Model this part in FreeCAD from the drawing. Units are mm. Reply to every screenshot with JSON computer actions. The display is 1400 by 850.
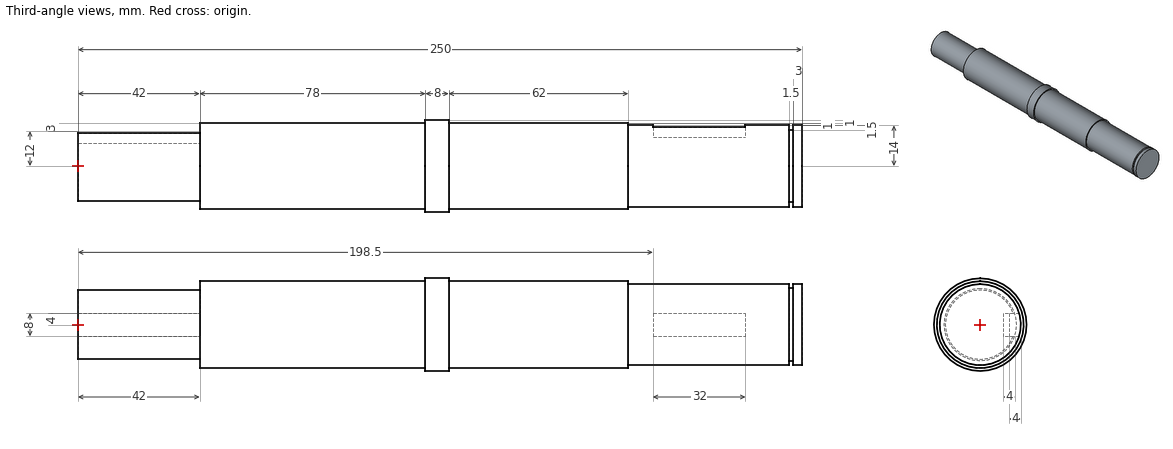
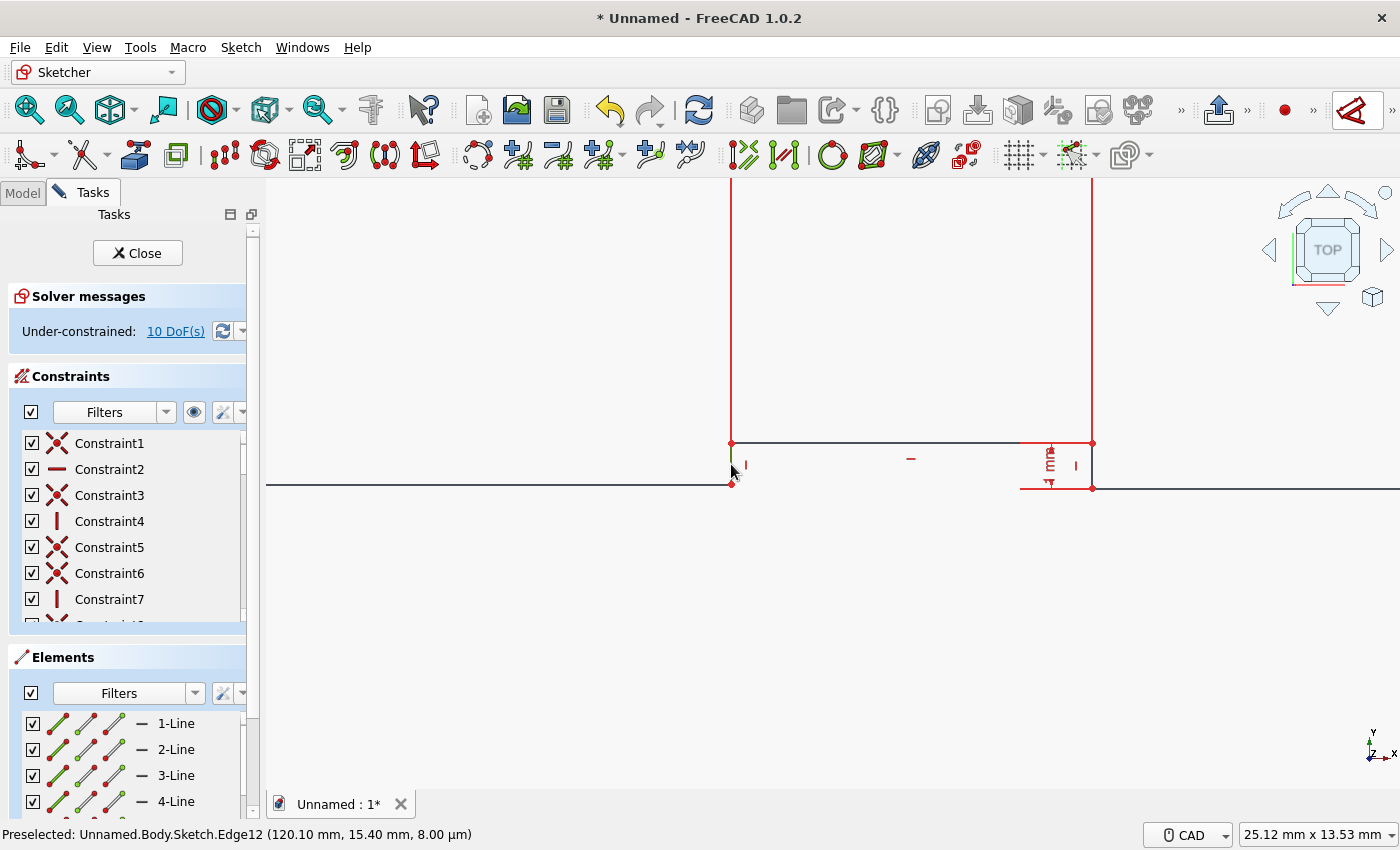
{"action": "left_click", "coordinate": [1378, 110]}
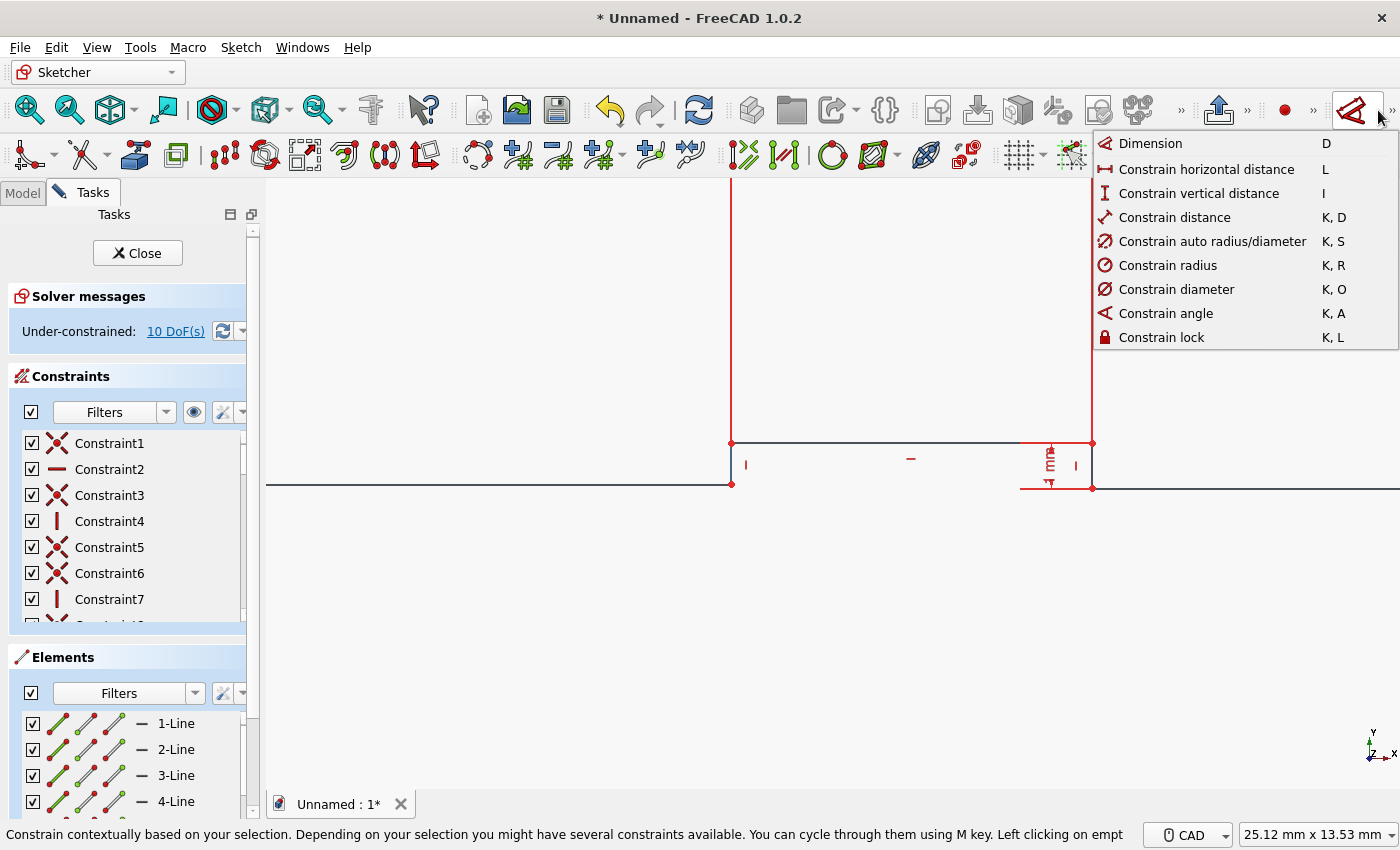
{"action": "left_click", "coordinate": [1246, 193]}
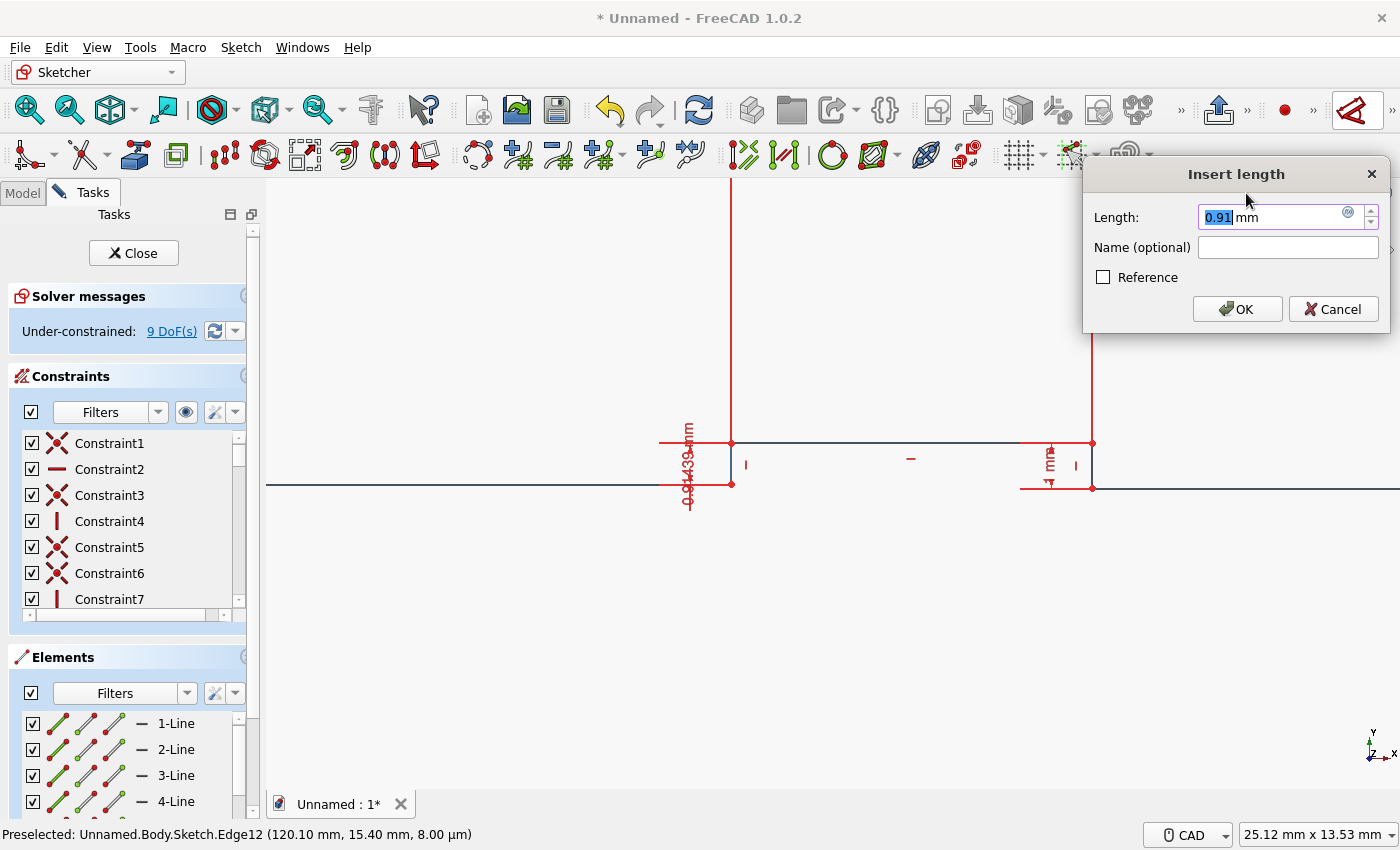
{"action": "type", "text": "1"}
{"action": "key", "text": "Return"}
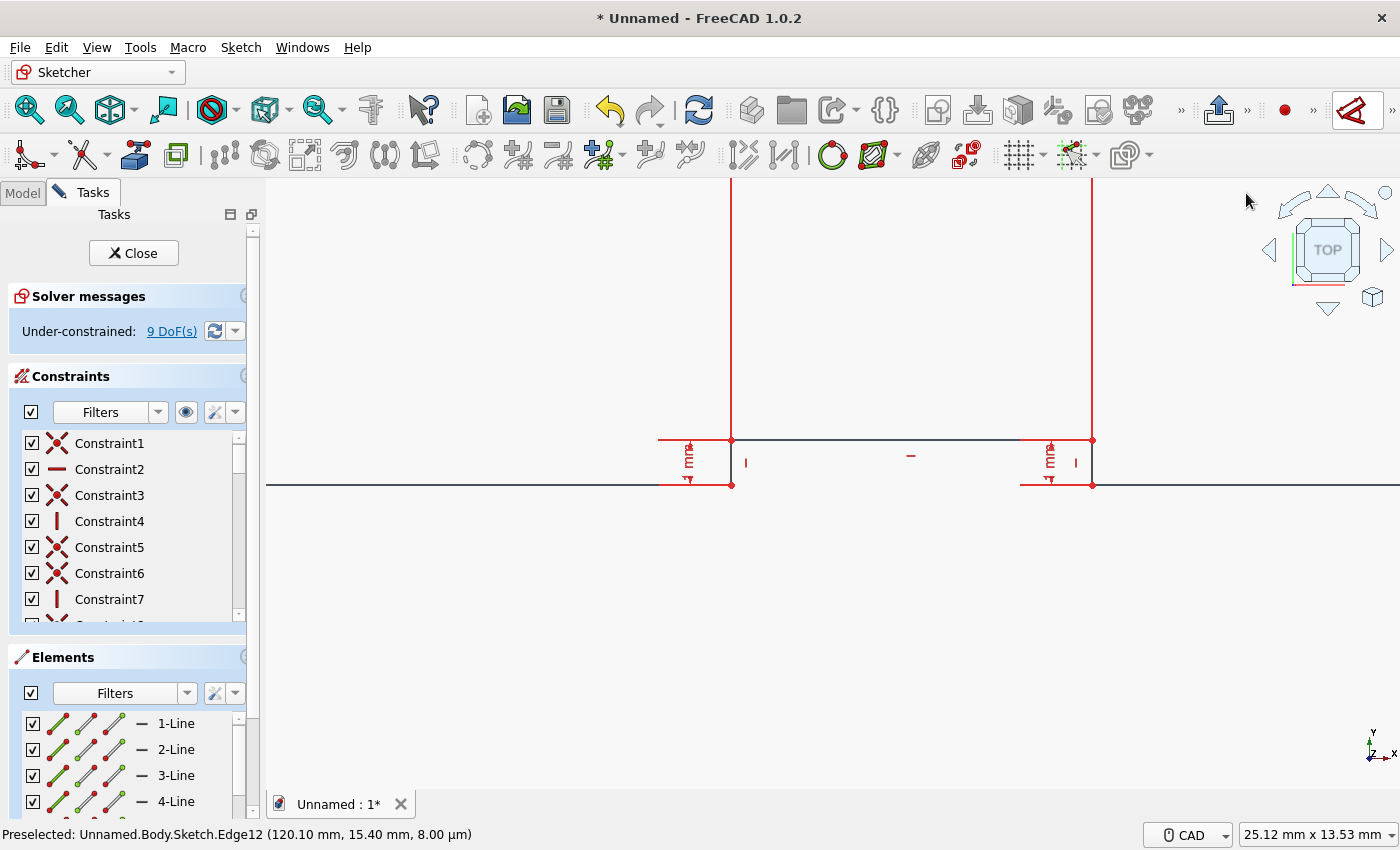
{"action": "scroll", "coordinate": [752, 463], "scroll_direction": "down", "scroll_amount": 14}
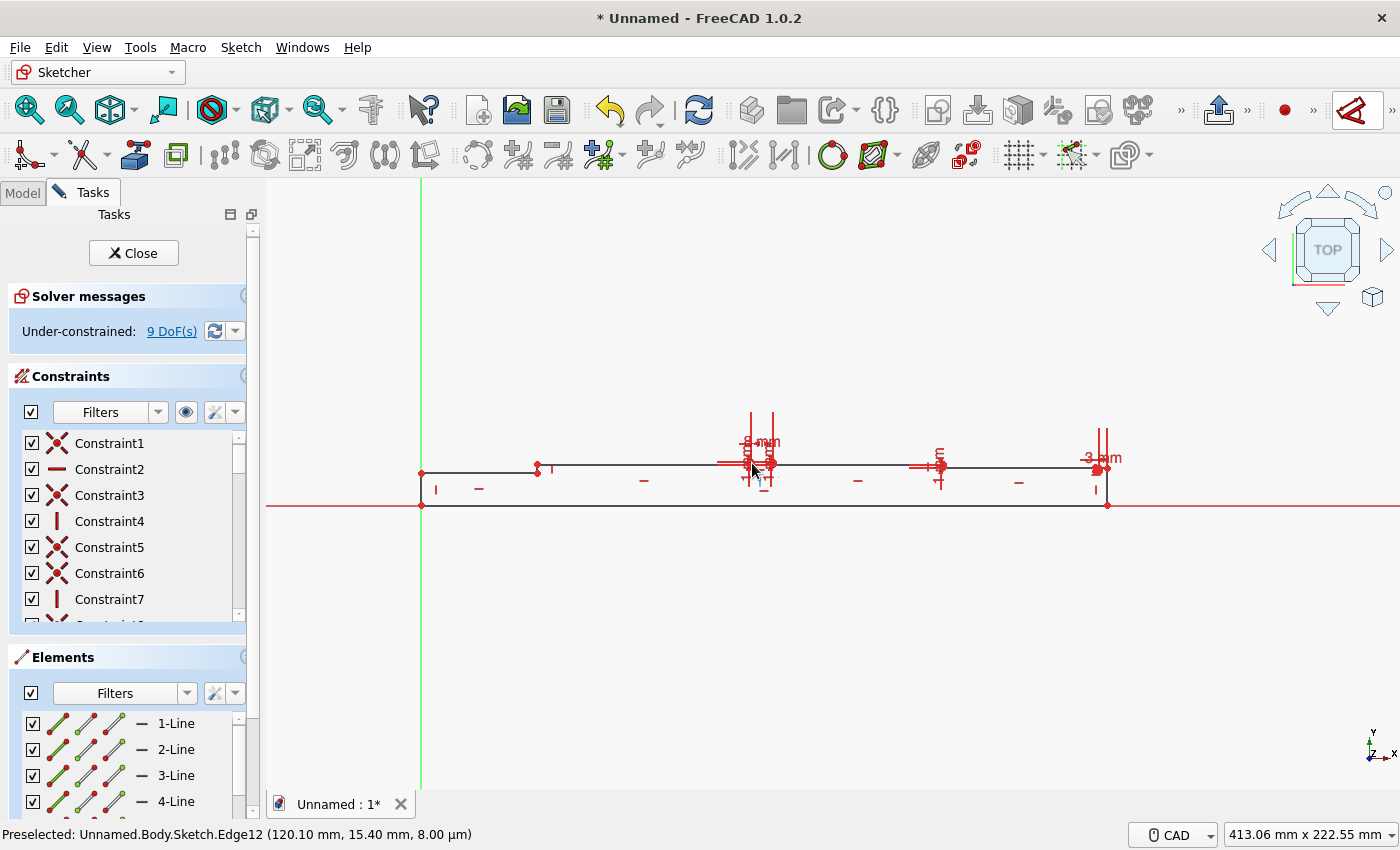
{"action": "scroll", "coordinate": [537, 467], "scroll_direction": "up", "scroll_amount": 9}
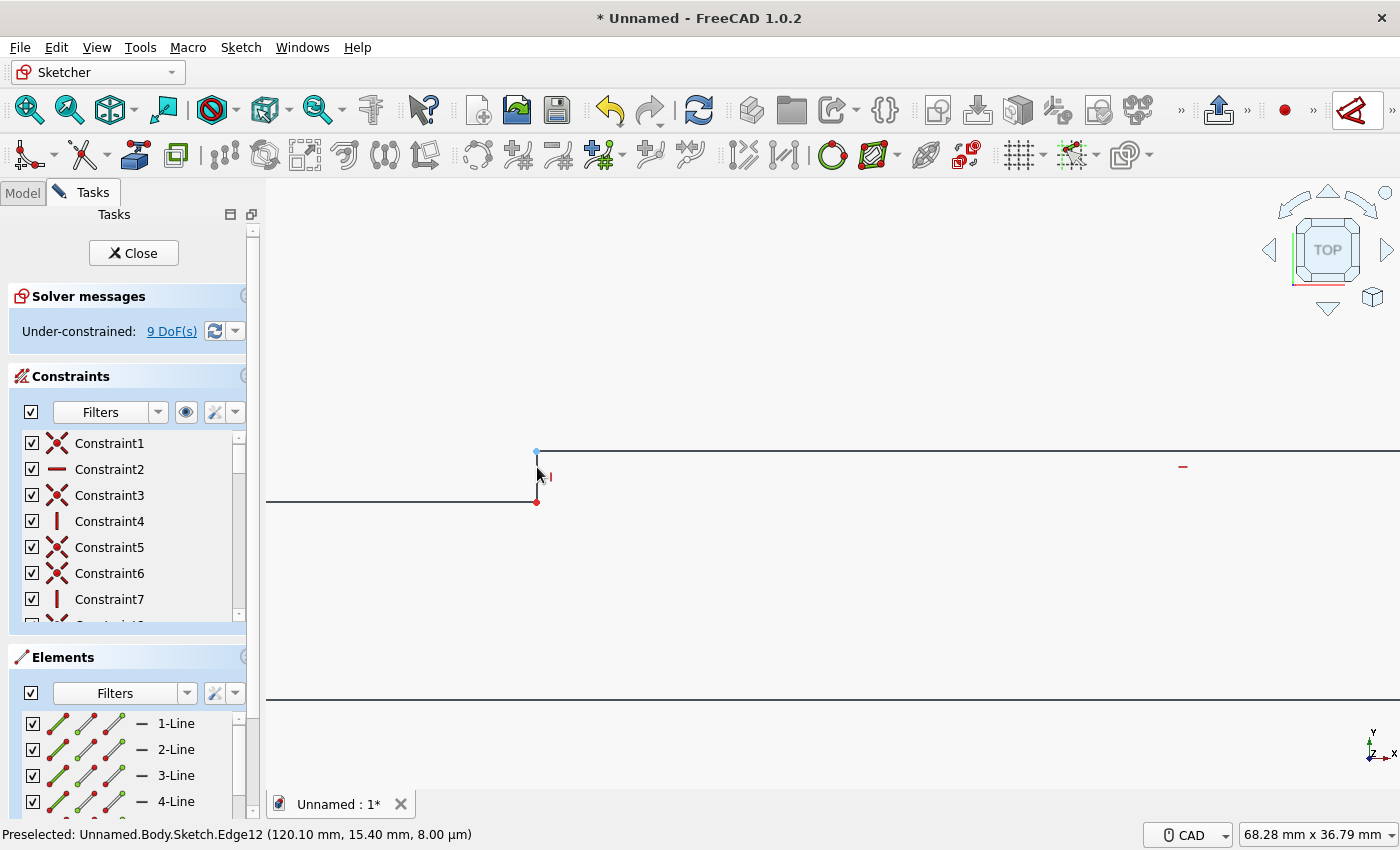
{"action": "left_click", "coordinate": [537, 466]}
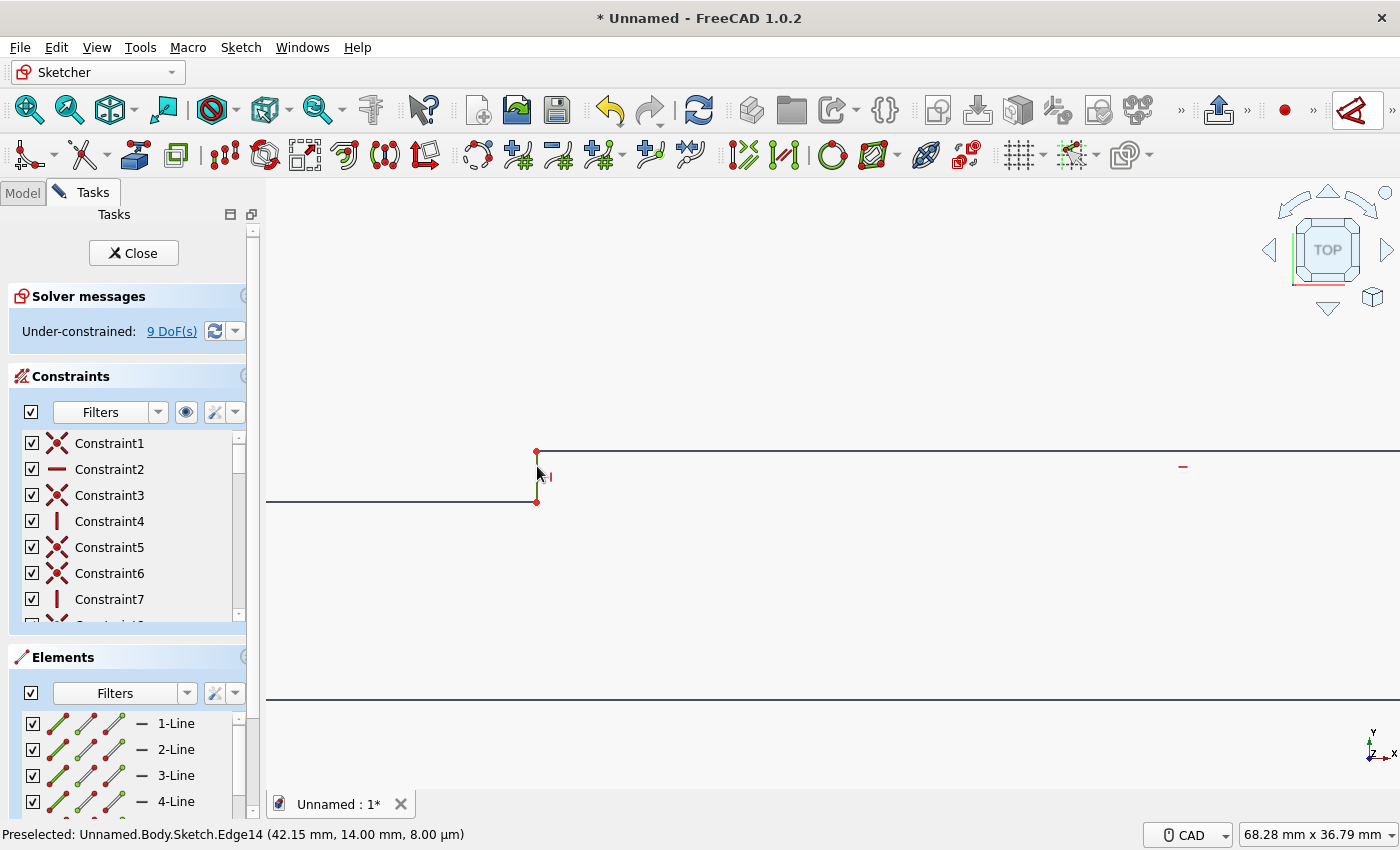
{"action": "left_click", "coordinate": [1378, 110]}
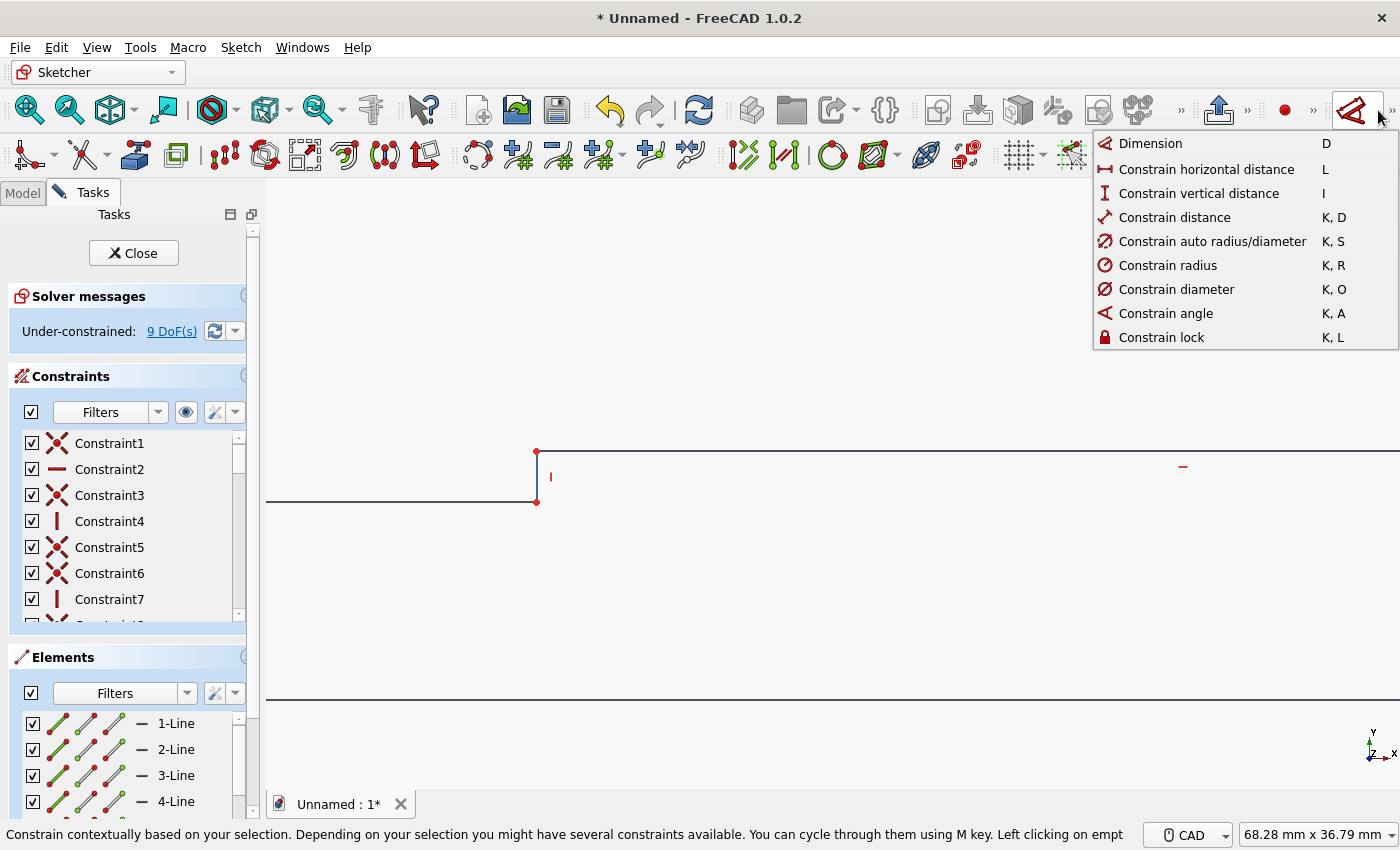
{"action": "left_click", "coordinate": [1246, 193]}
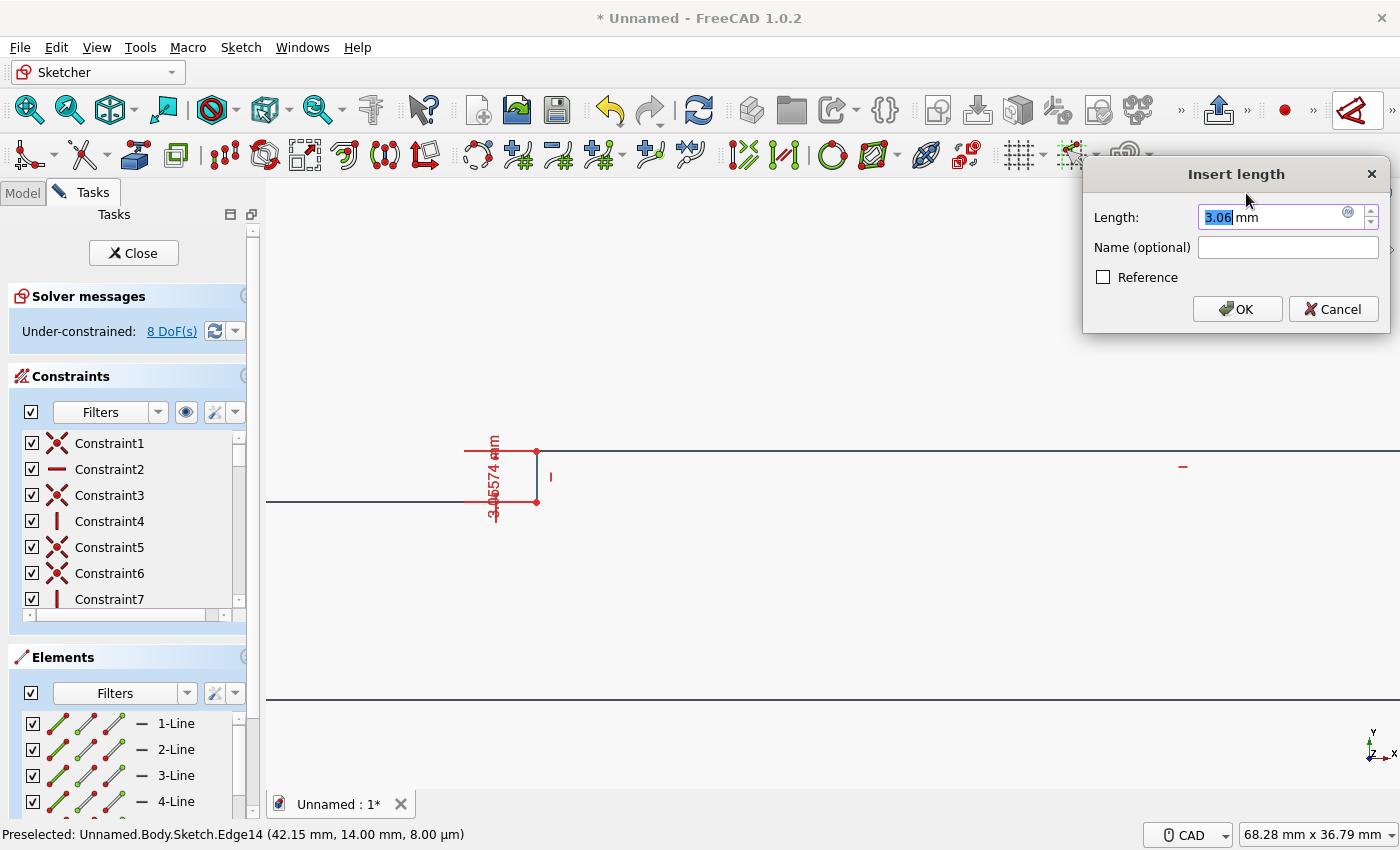
{"action": "type", "text": "3"}
{"action": "key", "text": "Return"}